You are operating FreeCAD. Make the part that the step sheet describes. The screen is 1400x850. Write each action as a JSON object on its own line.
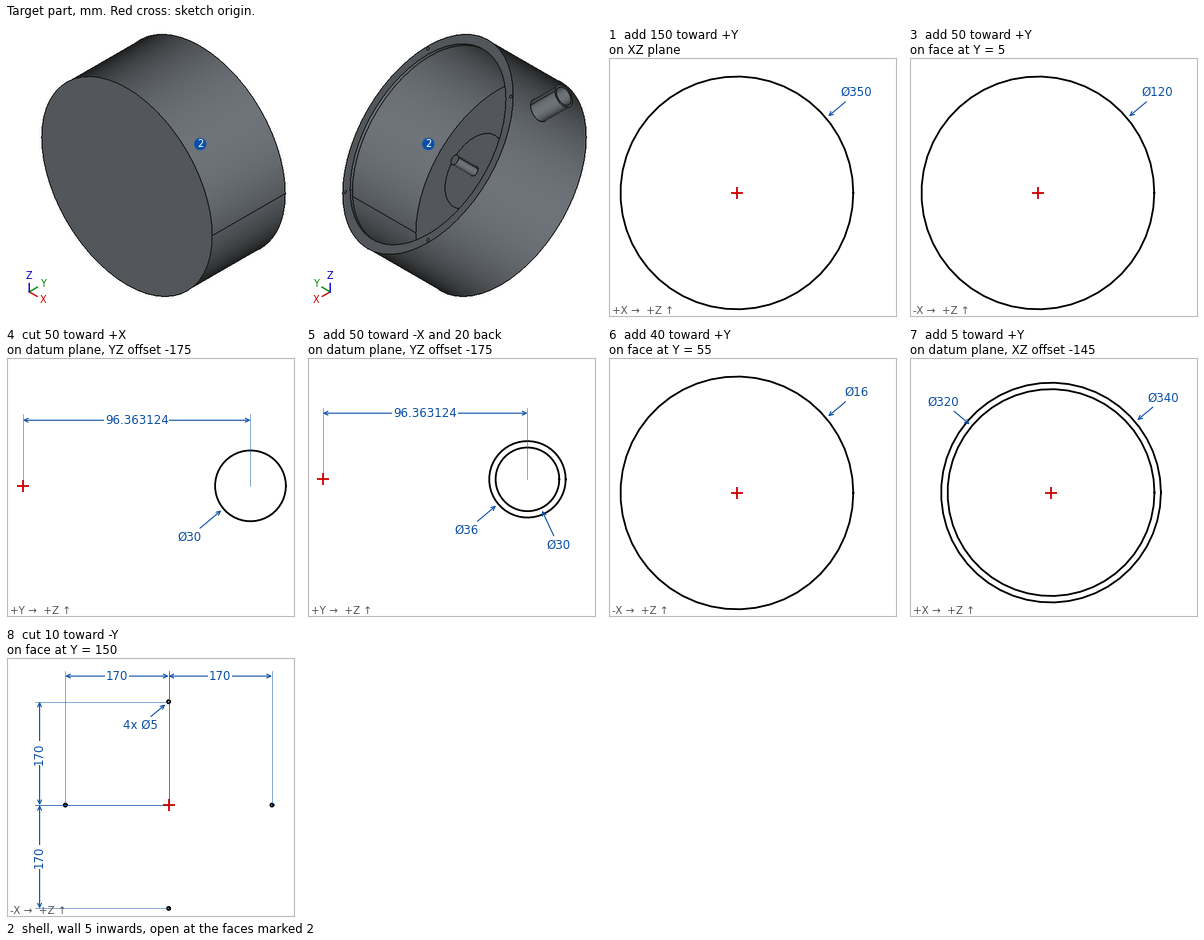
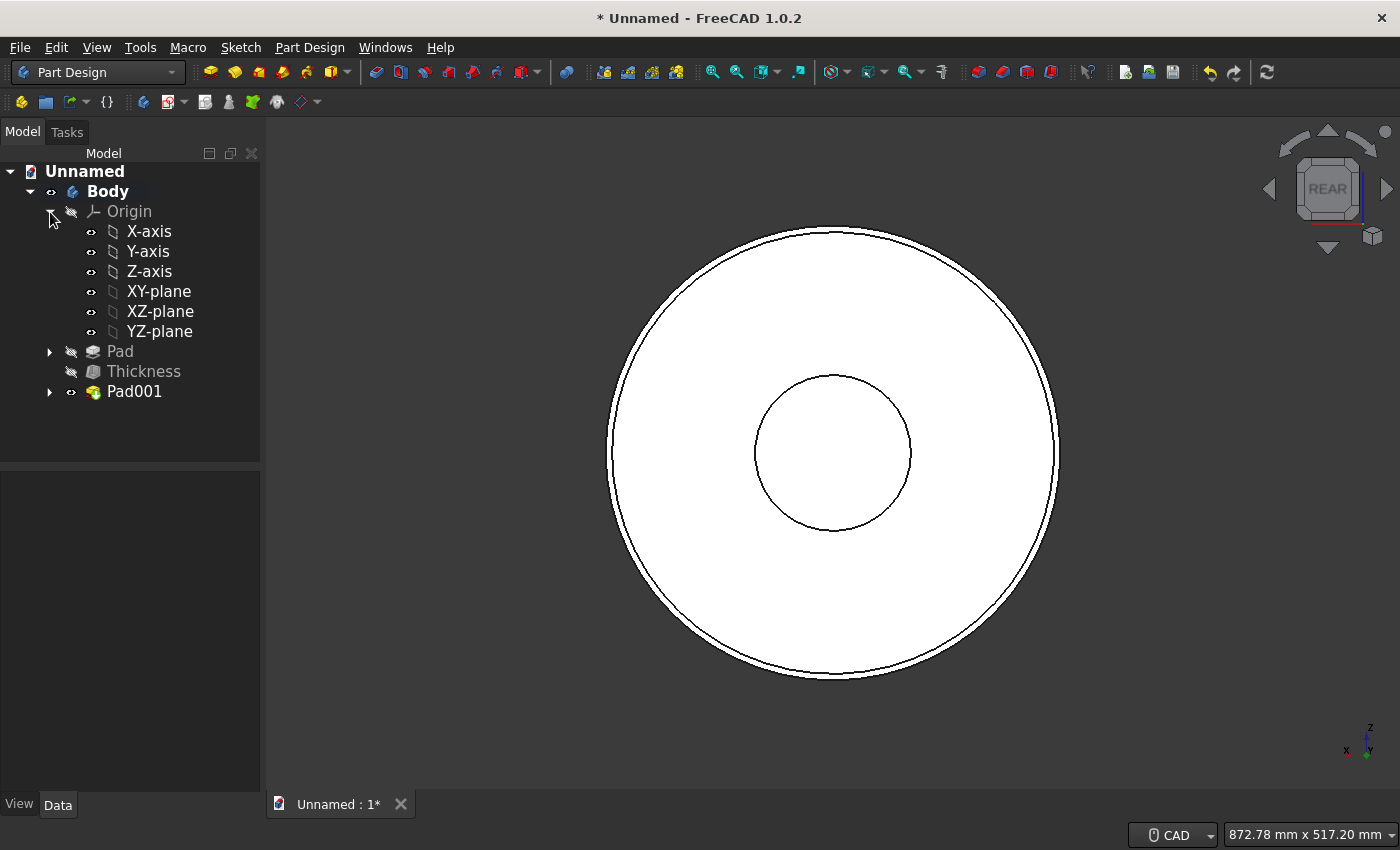
{"action": "left_click", "coordinate": [136, 332]}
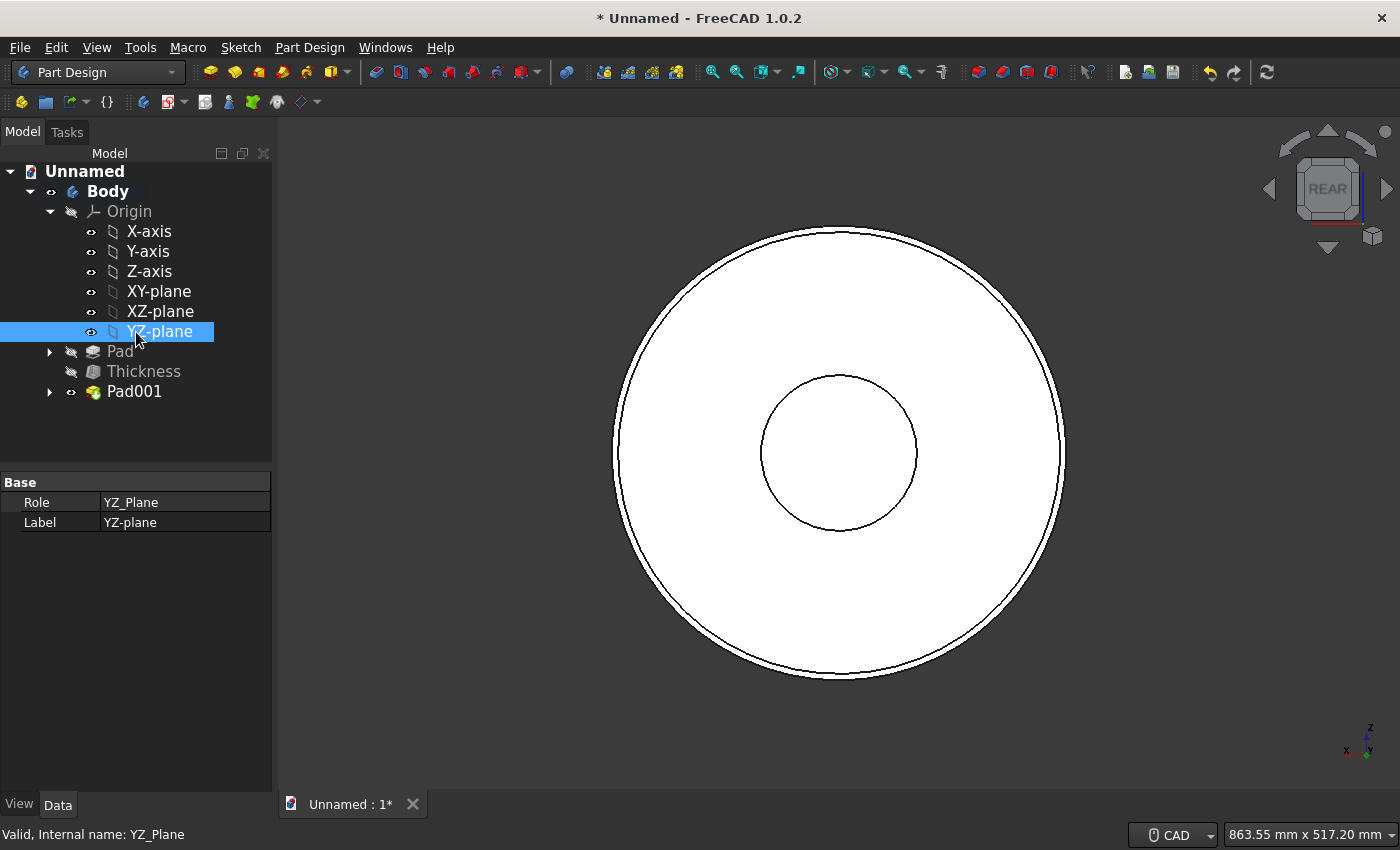
{"action": "left_click", "coordinate": [302, 102]}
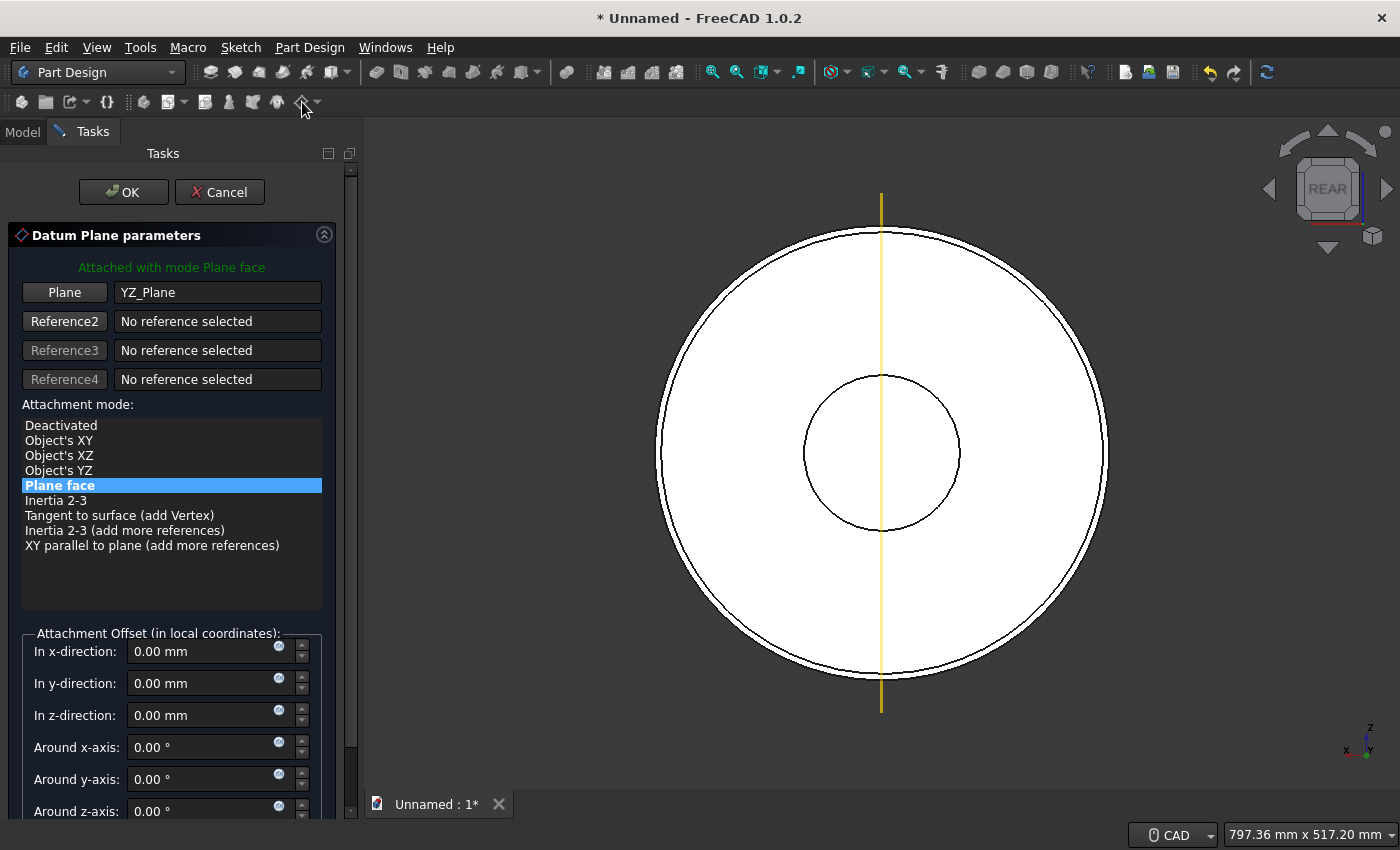
{"action": "triple_click", "coordinate": [210, 715]}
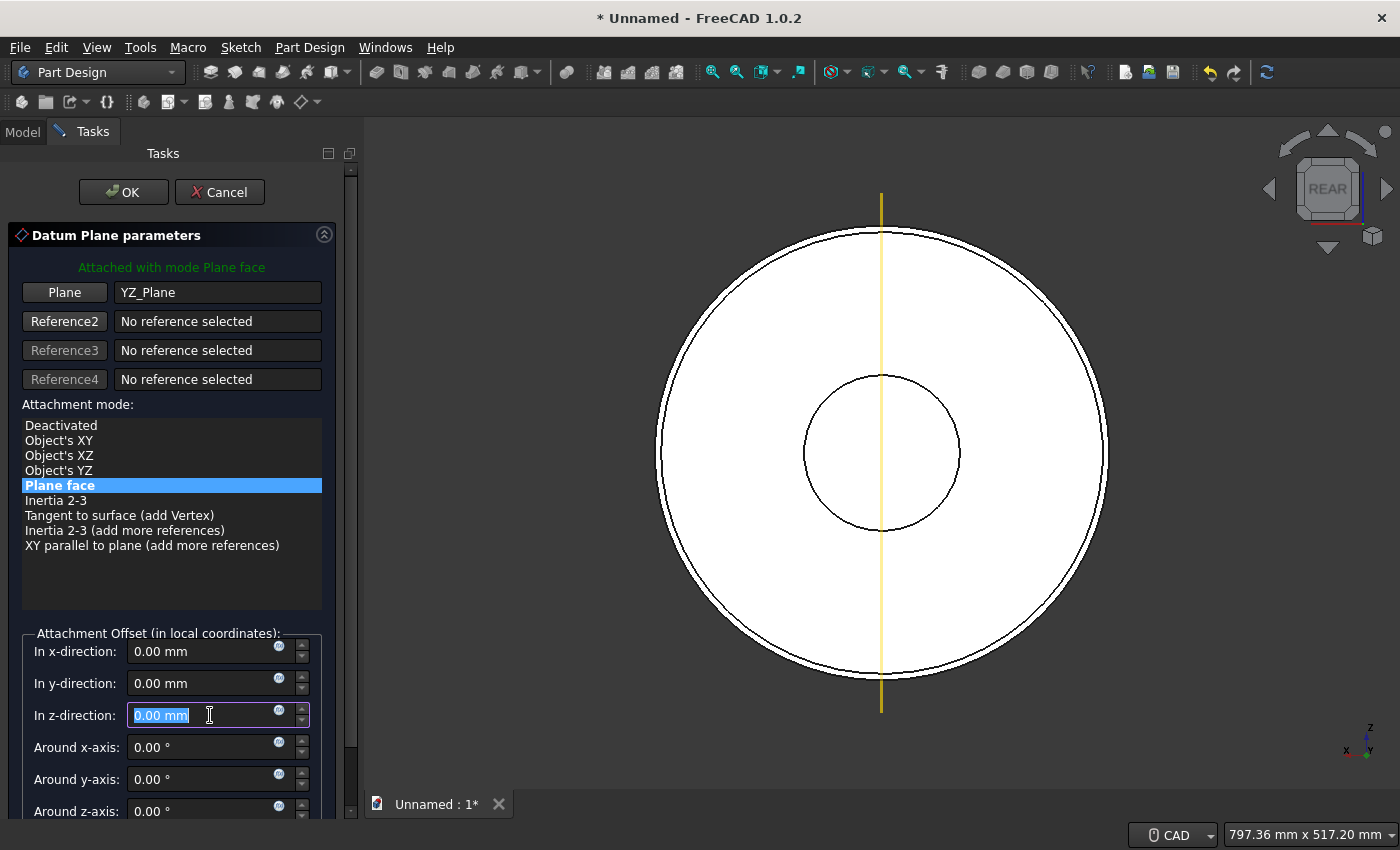
{"action": "type", "text": "-175"}
{"action": "key", "text": "Tab"}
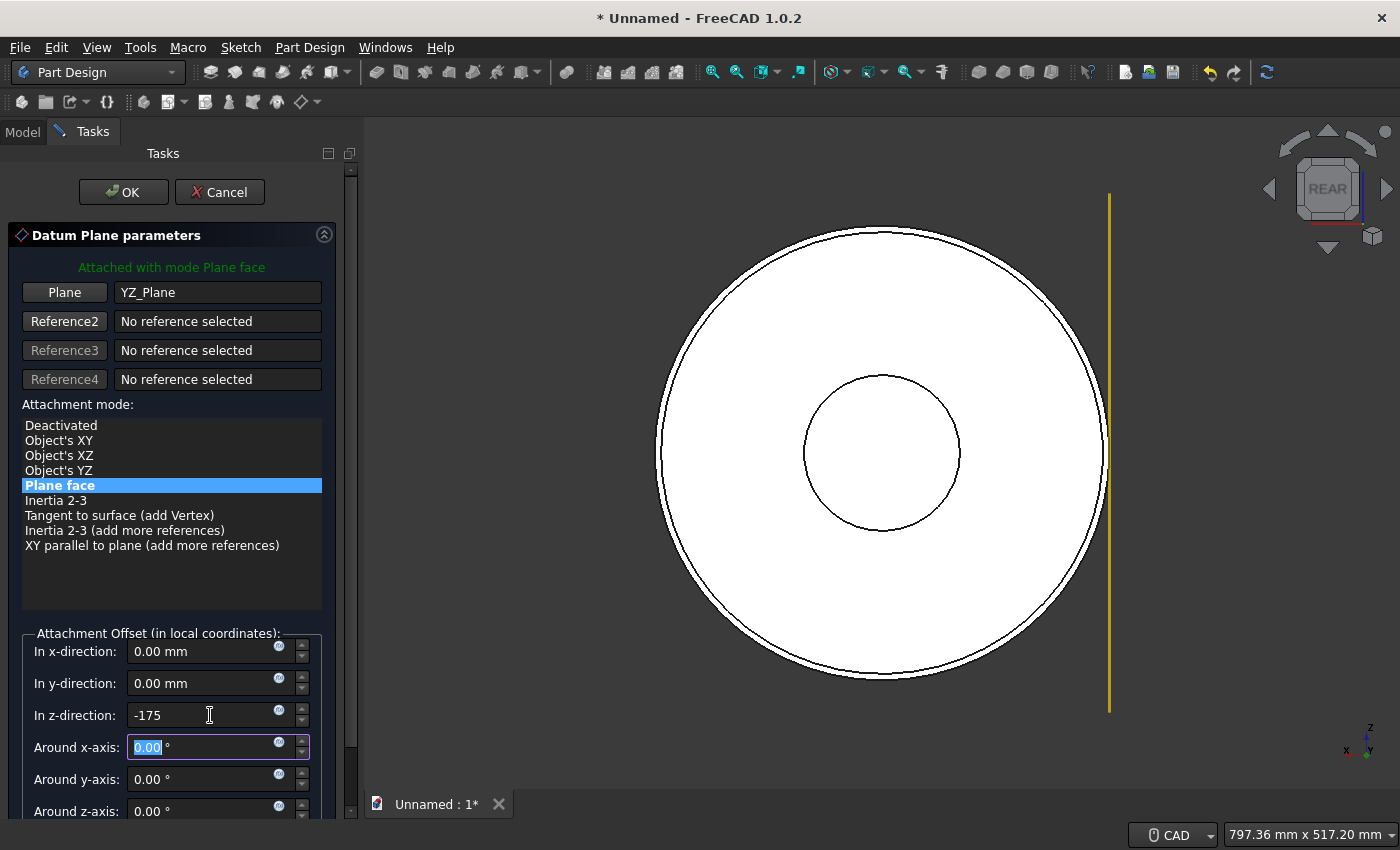
{"action": "left_click", "coordinate": [124, 192]}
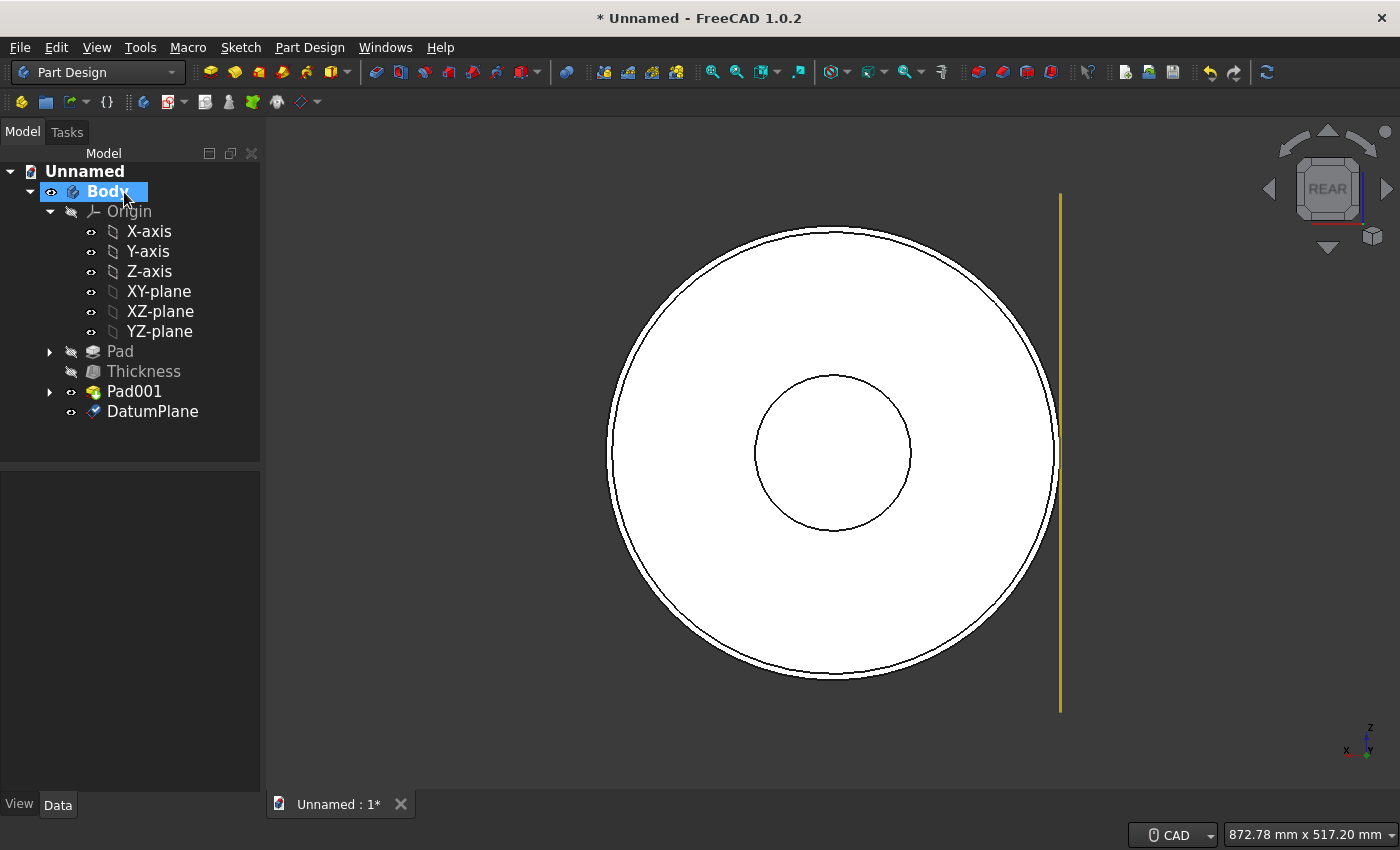
{"action": "left_click", "coordinate": [116, 412]}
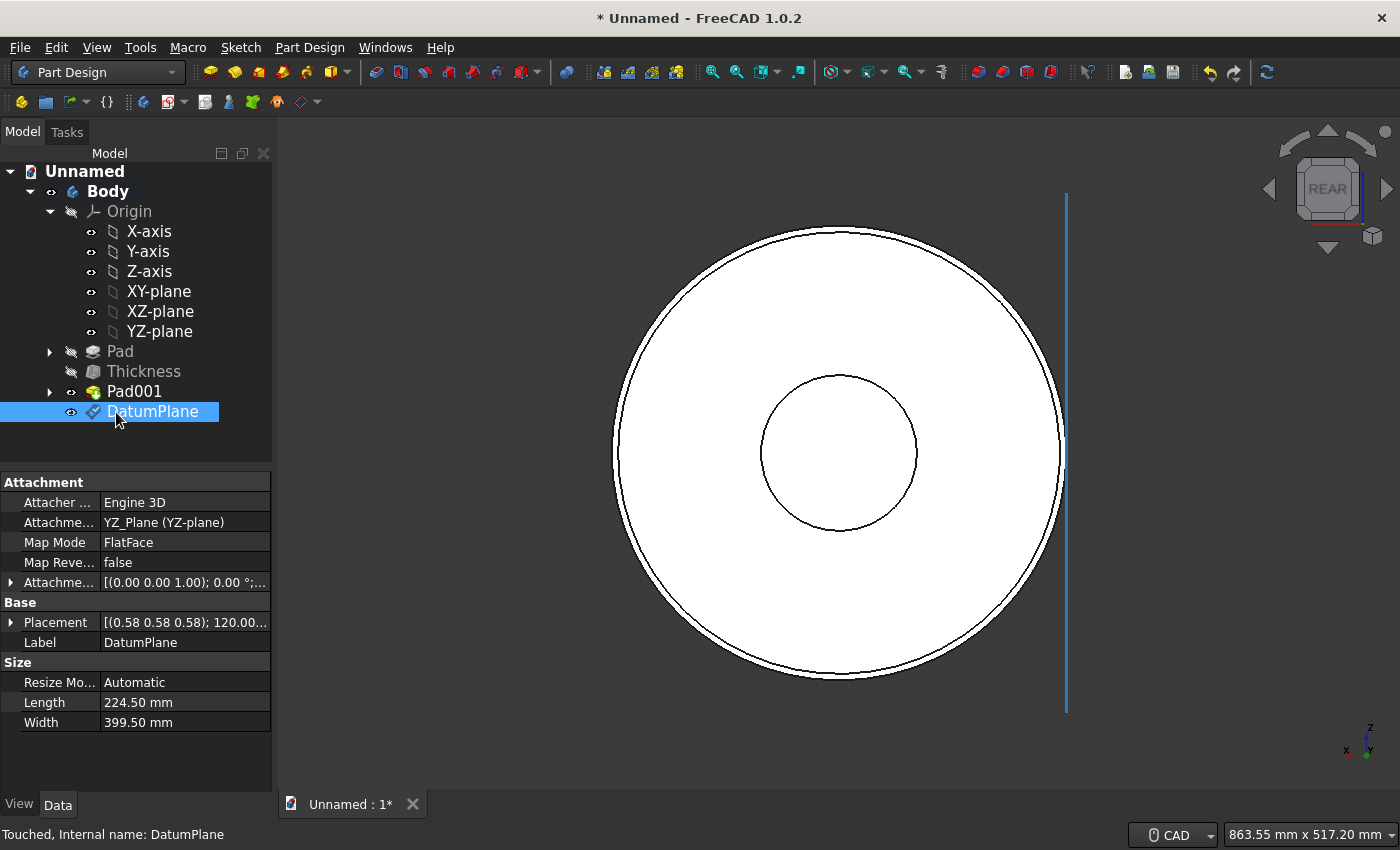
{"action": "left_click", "coordinate": [168, 102]}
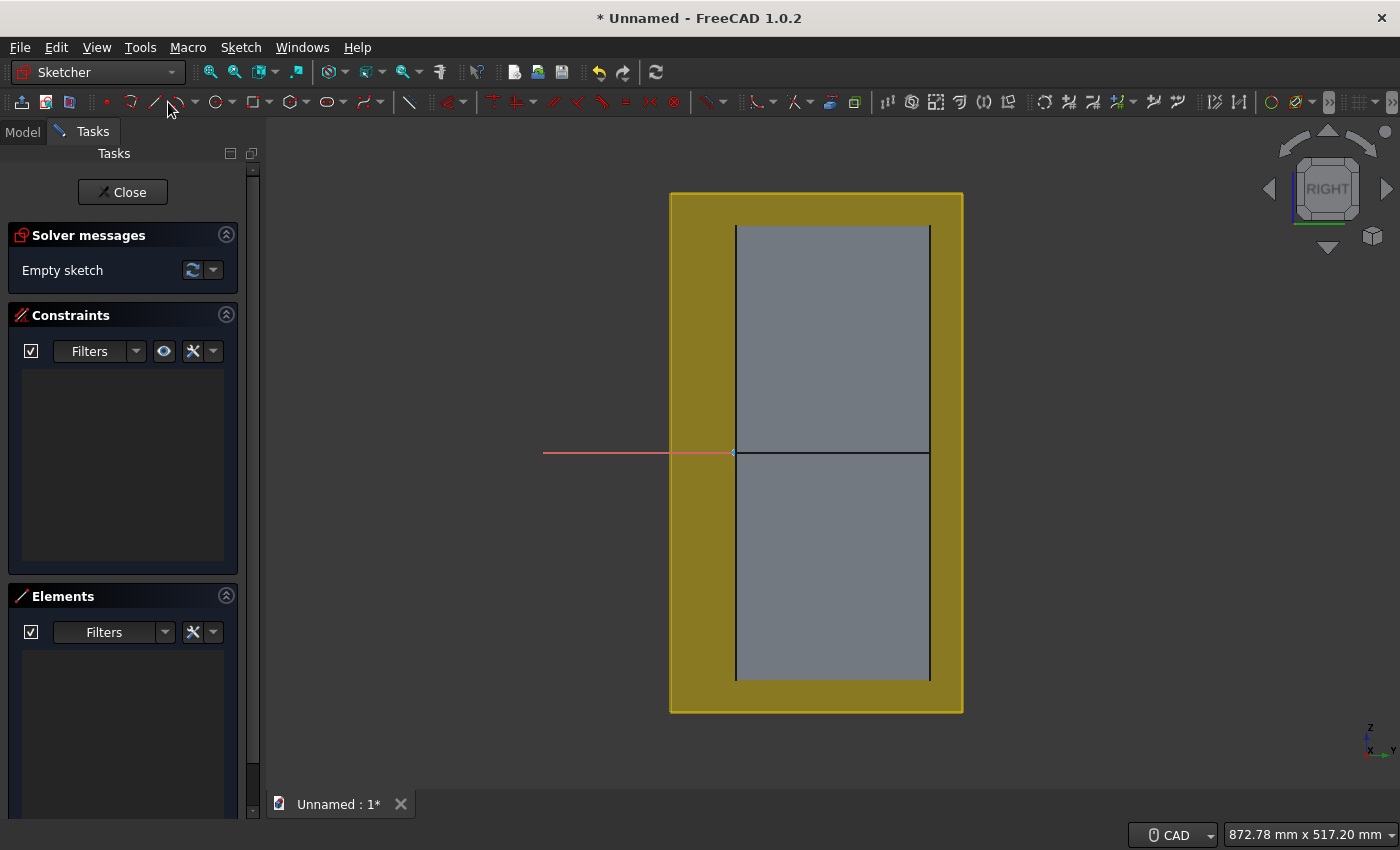
{"action": "left_click", "coordinate": [70, 102]}